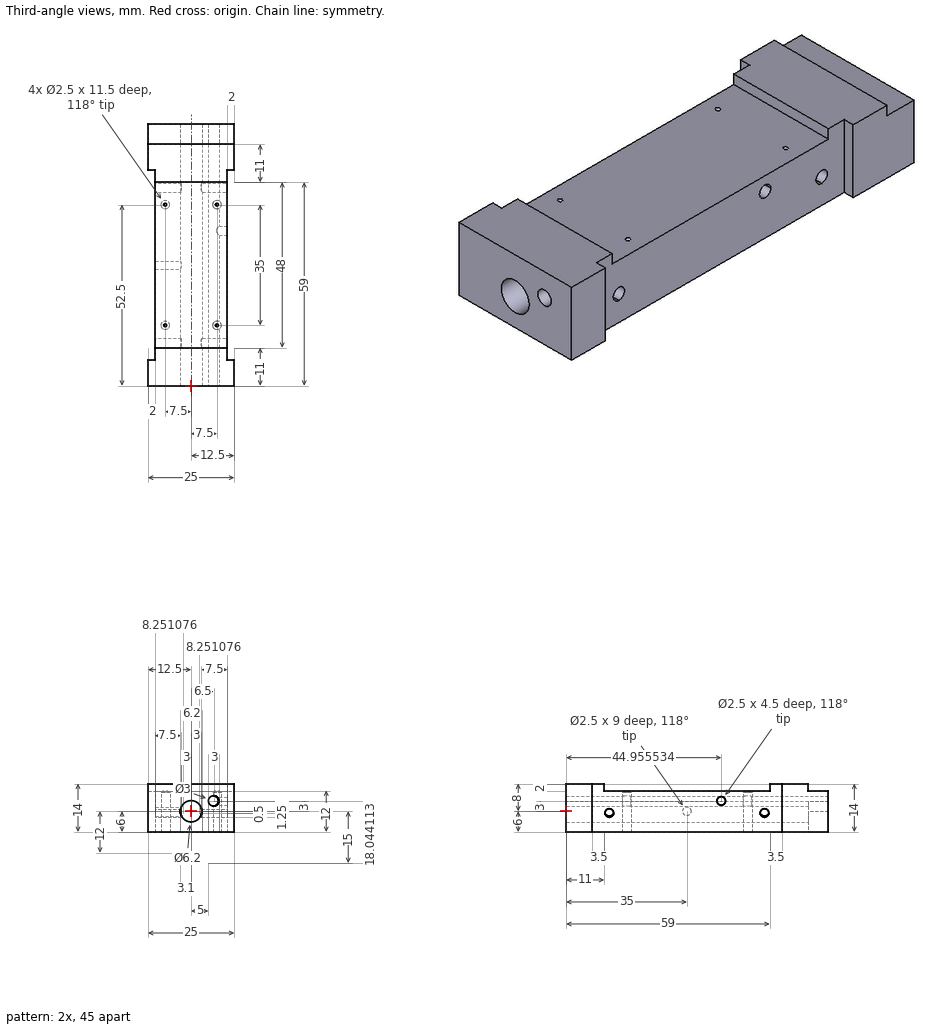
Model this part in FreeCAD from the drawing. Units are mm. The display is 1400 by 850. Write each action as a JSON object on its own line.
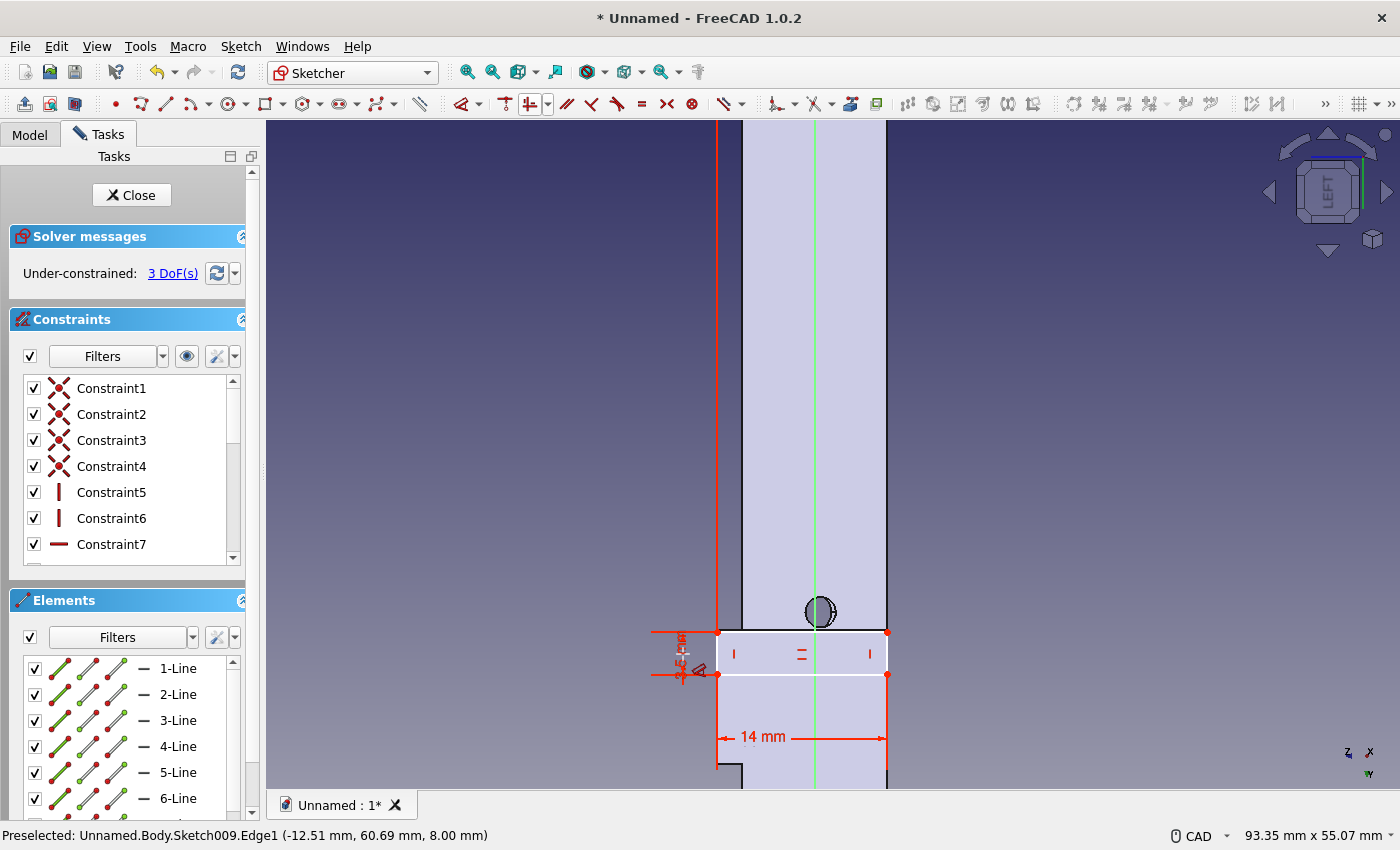
{"action": "scroll", "coordinate": [718, 650], "scroll_direction": "down", "scroll_amount": 3}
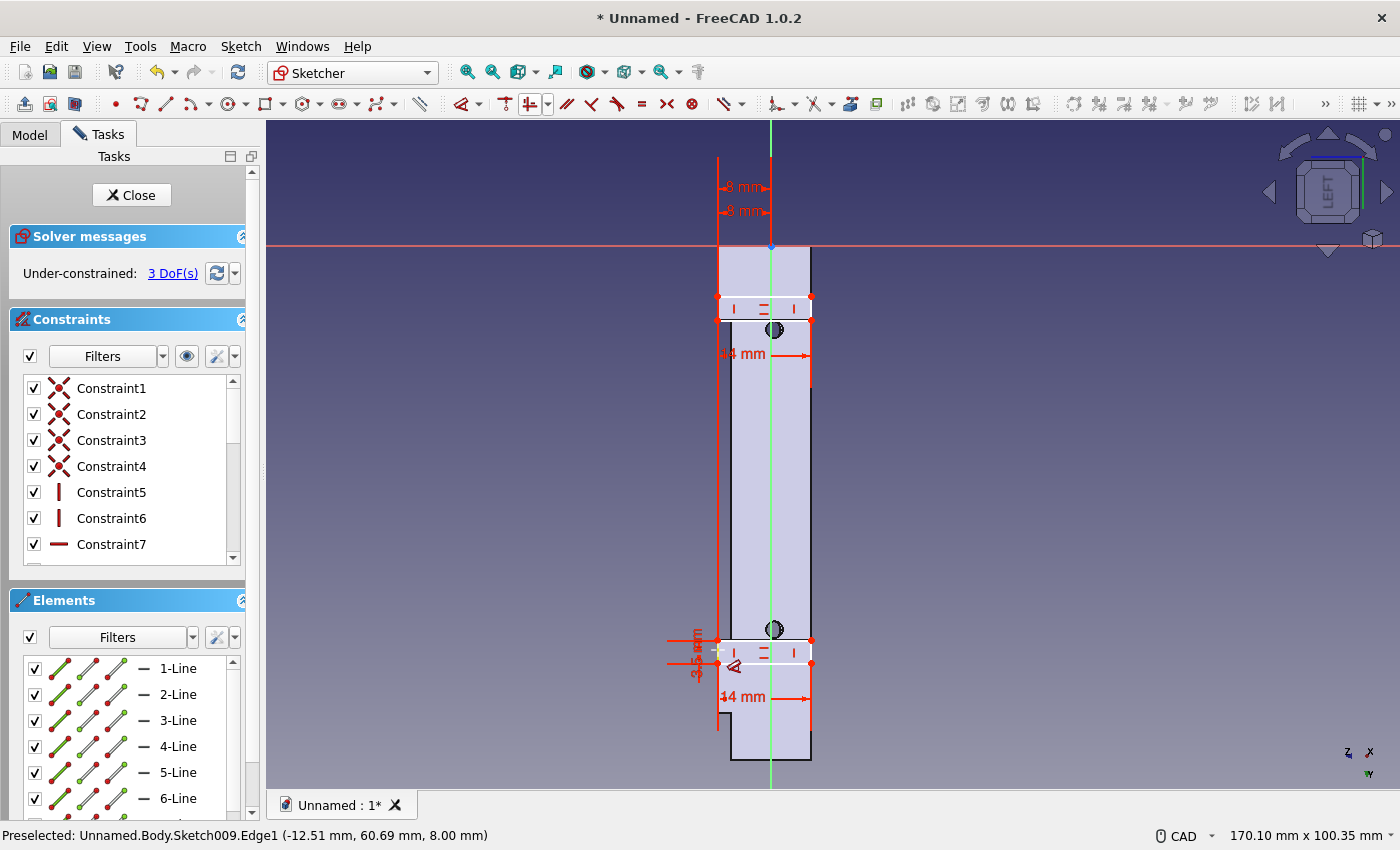
{"action": "scroll", "coordinate": [718, 304], "scroll_direction": "up", "scroll_amount": 4}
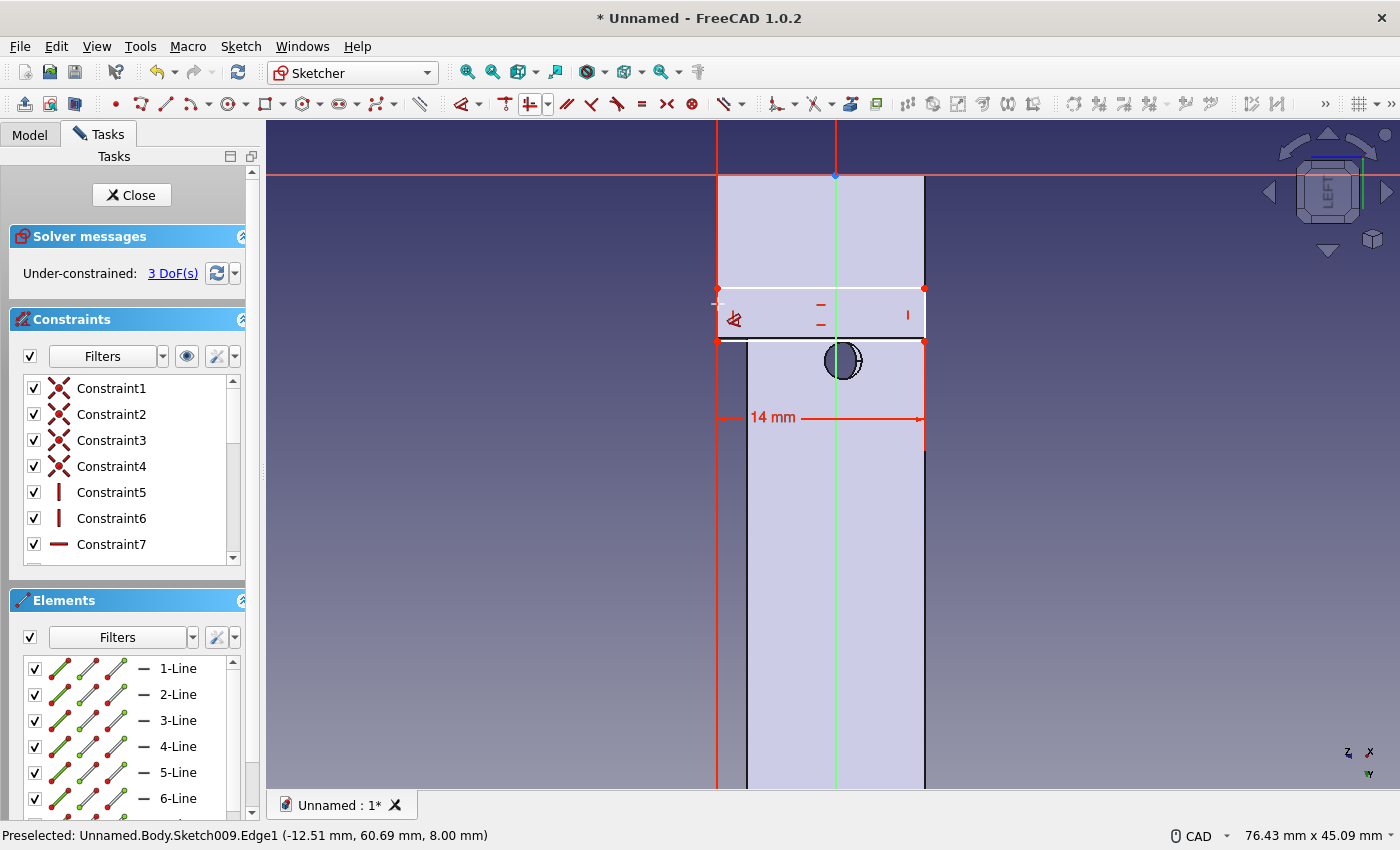
{"action": "left_click", "coordinate": [717, 304]}
{"action": "left_click", "coordinate": [683, 315]}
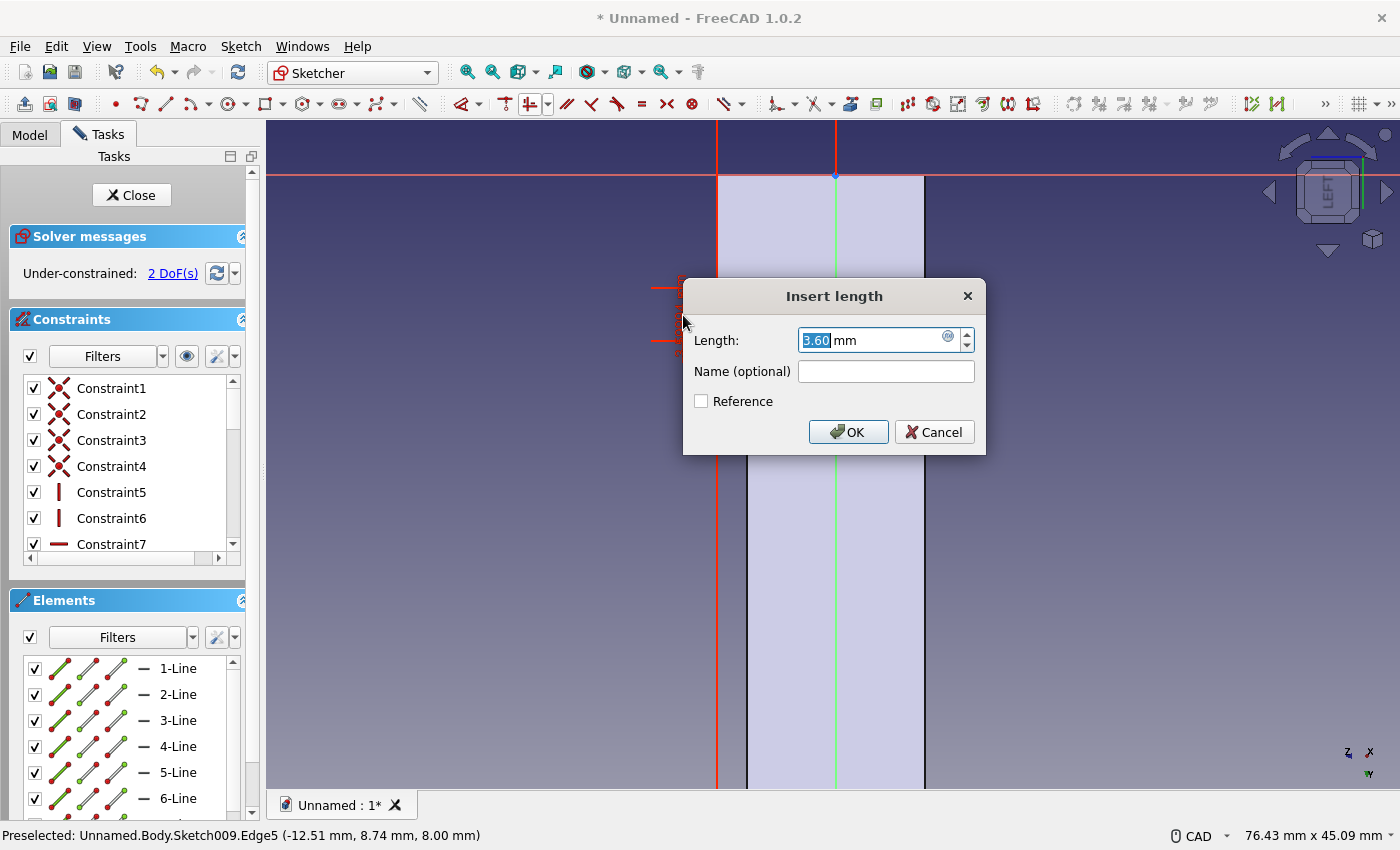
{"action": "type", "text": "3.5"}
{"action": "key", "text": "Return"}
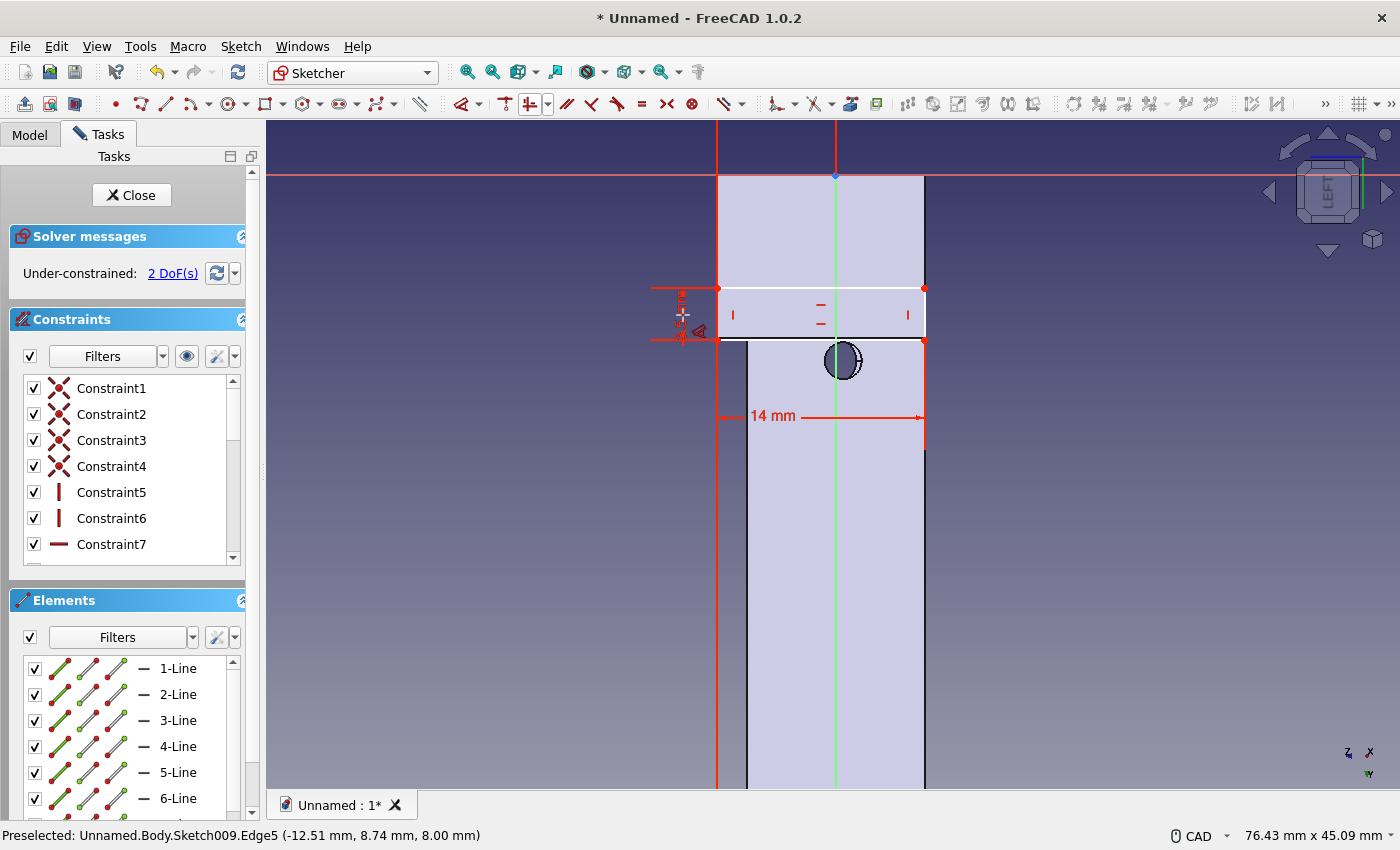
{"action": "scroll", "coordinate": [718, 304], "scroll_direction": "down", "scroll_amount": 4}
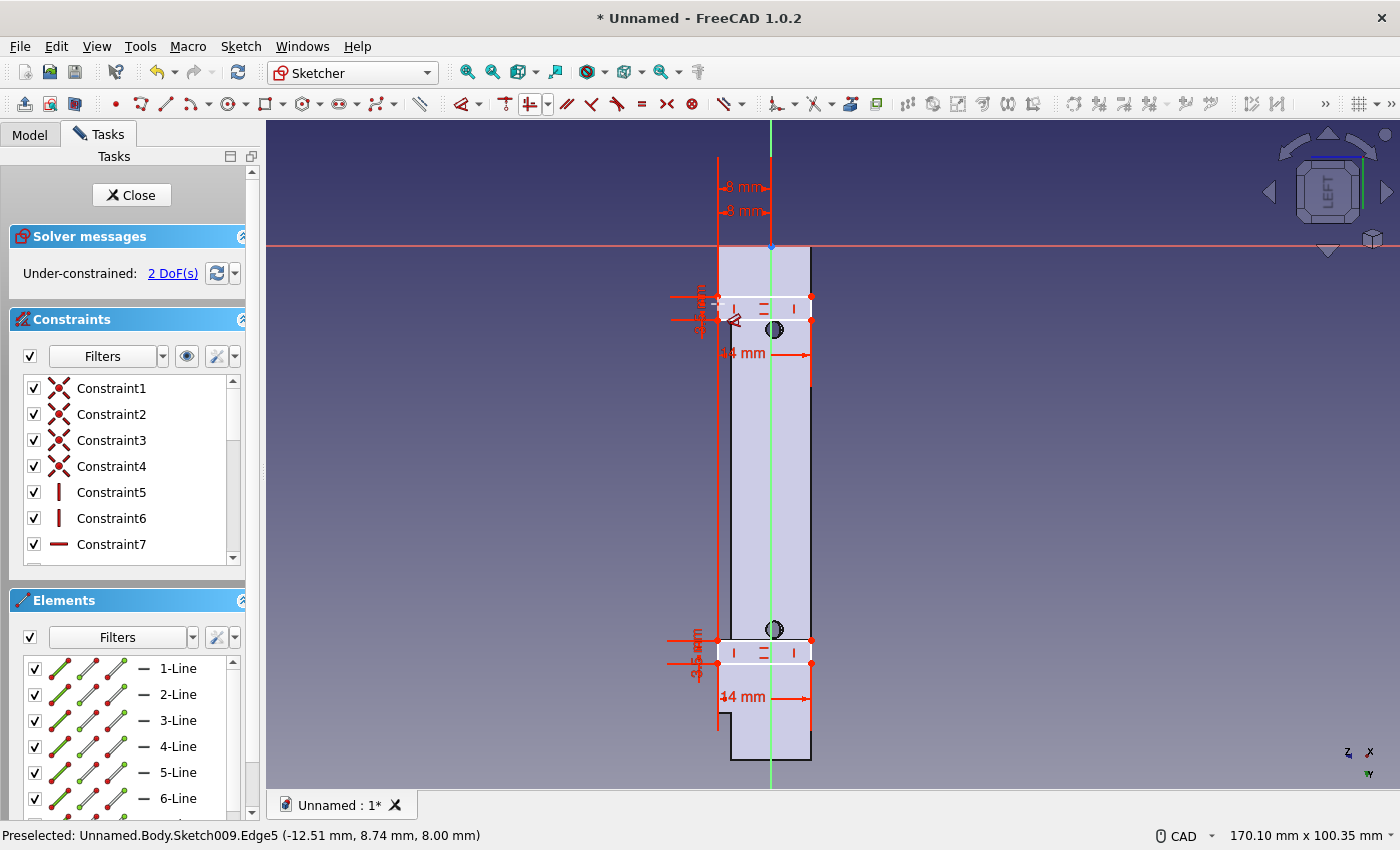
{"action": "left_click", "coordinate": [718, 641]}
{"action": "left_click", "coordinate": [684, 443]}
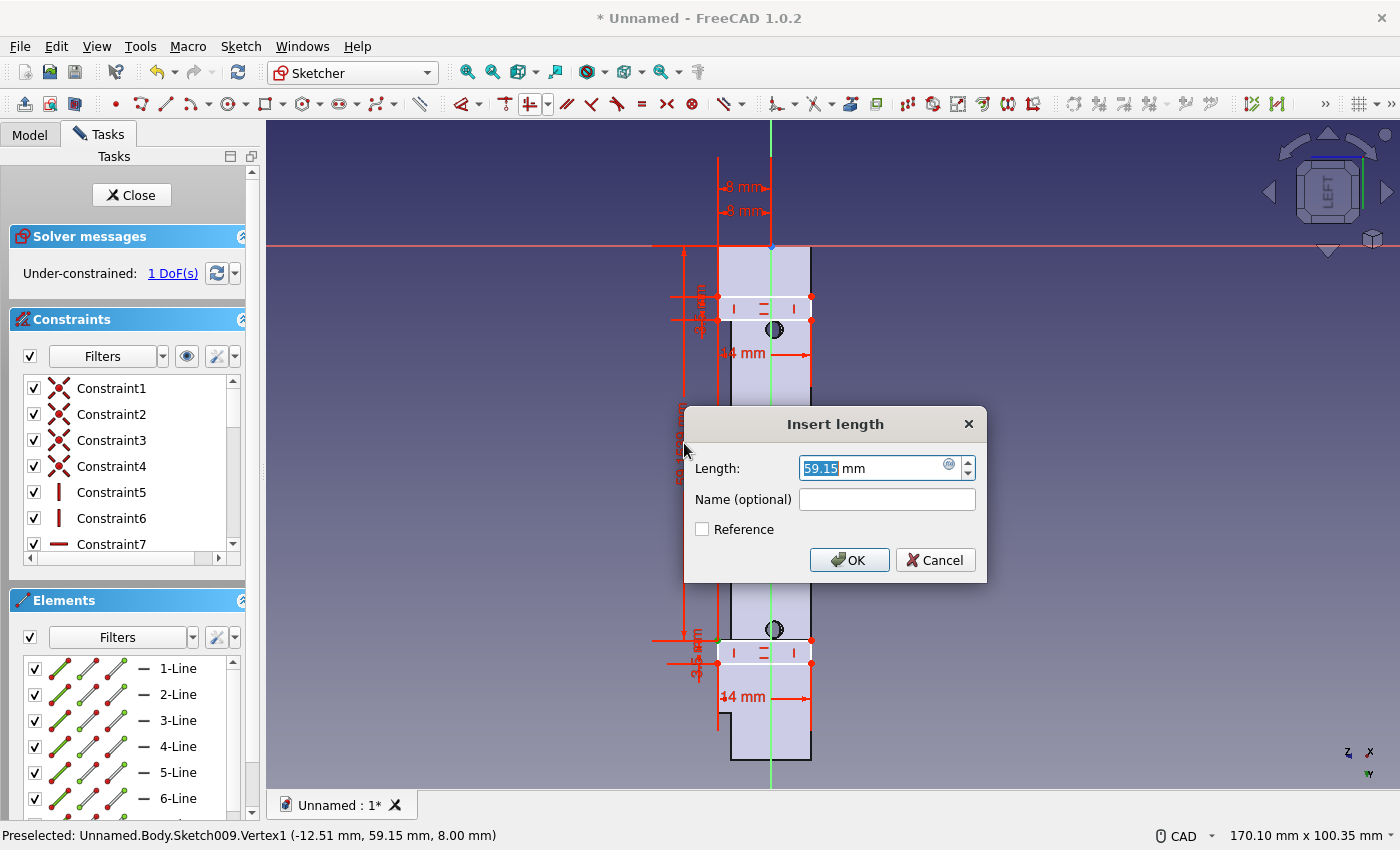
{"action": "type", "text": "59"}
{"action": "key", "text": "Return"}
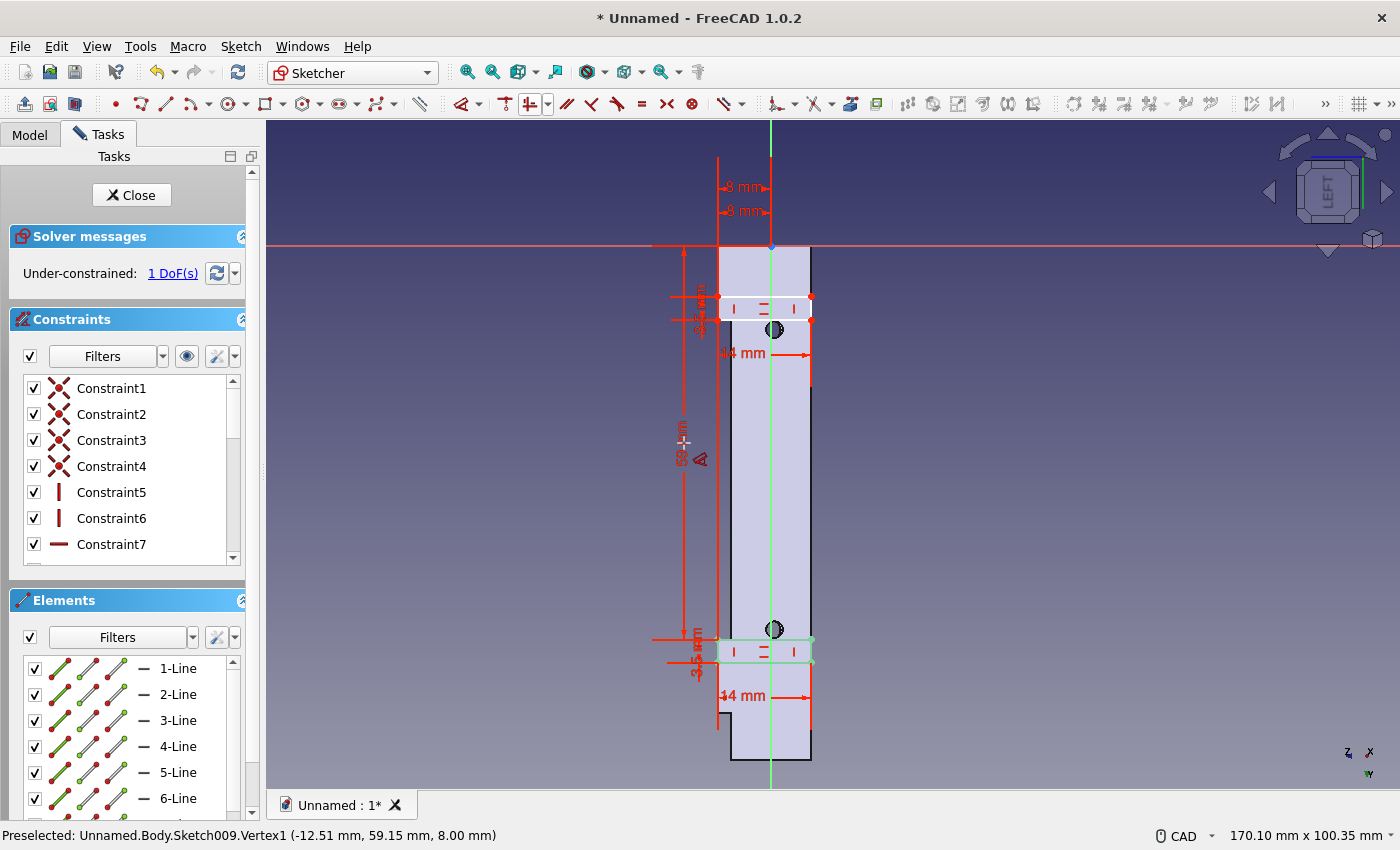
{"action": "left_click", "coordinate": [718, 320]}
{"action": "left_click", "coordinate": [684, 283]}